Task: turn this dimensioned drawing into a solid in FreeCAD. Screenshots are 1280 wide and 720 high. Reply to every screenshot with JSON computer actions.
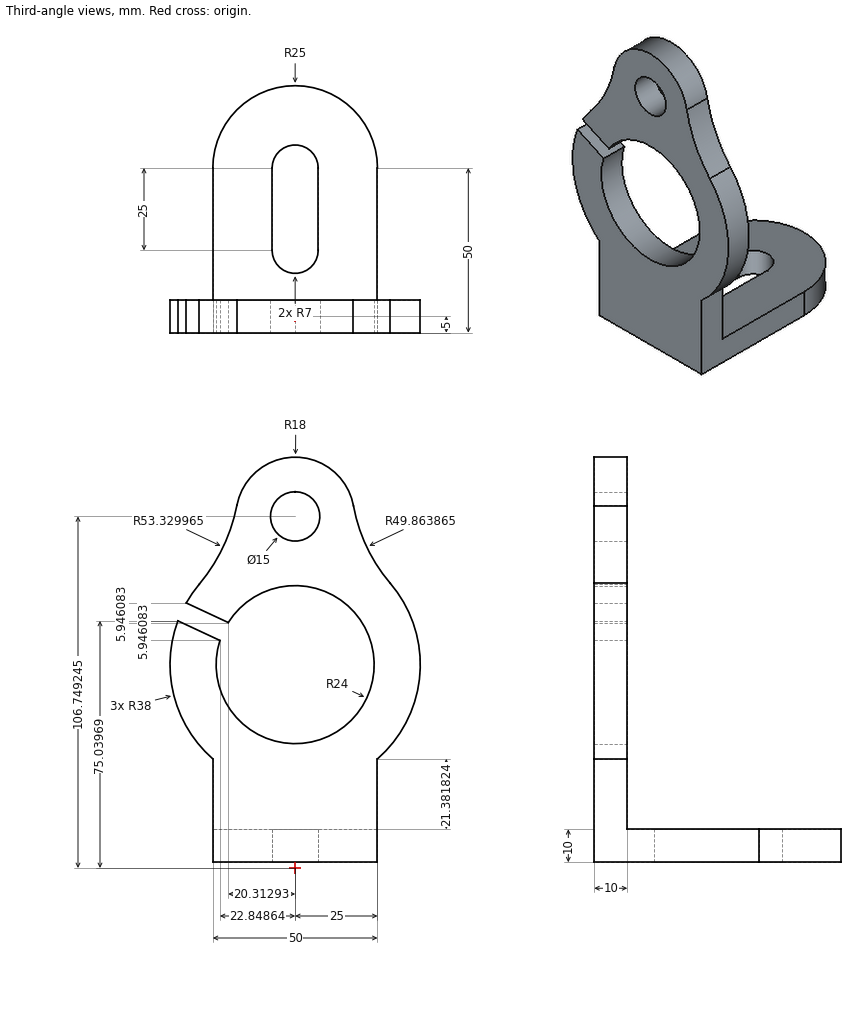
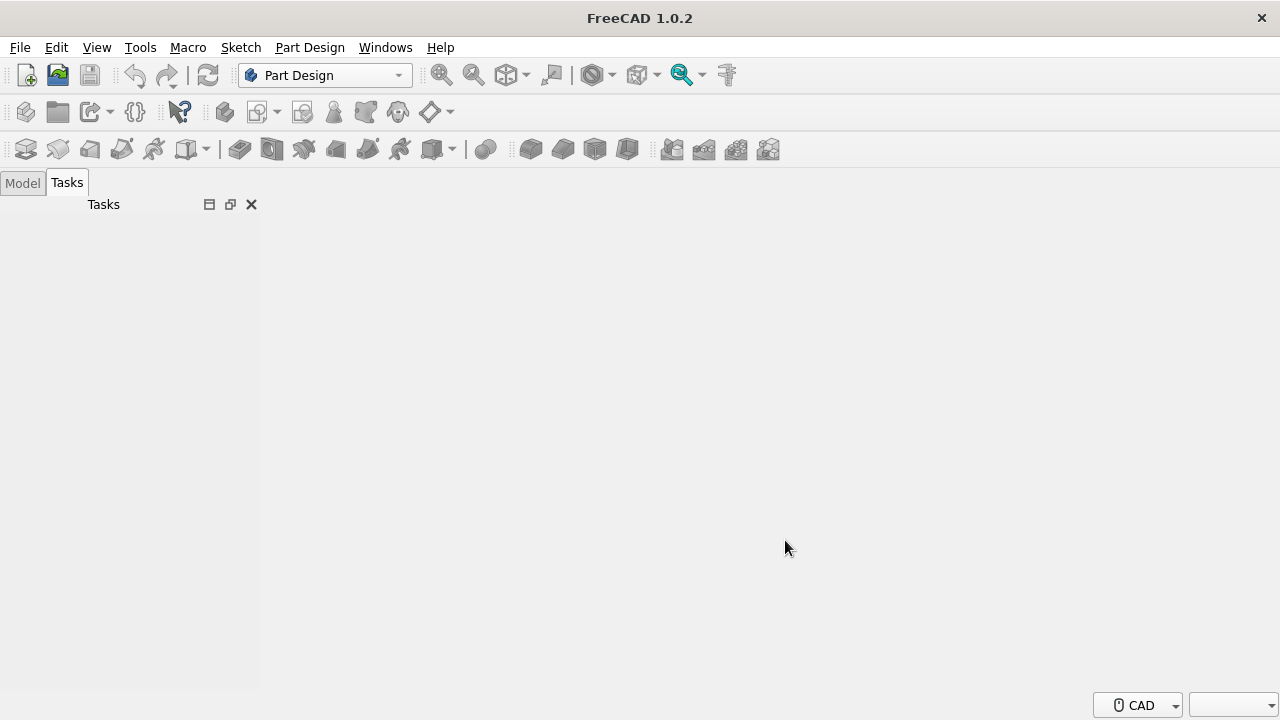
{"action": "left_click", "coordinate": [26, 76]}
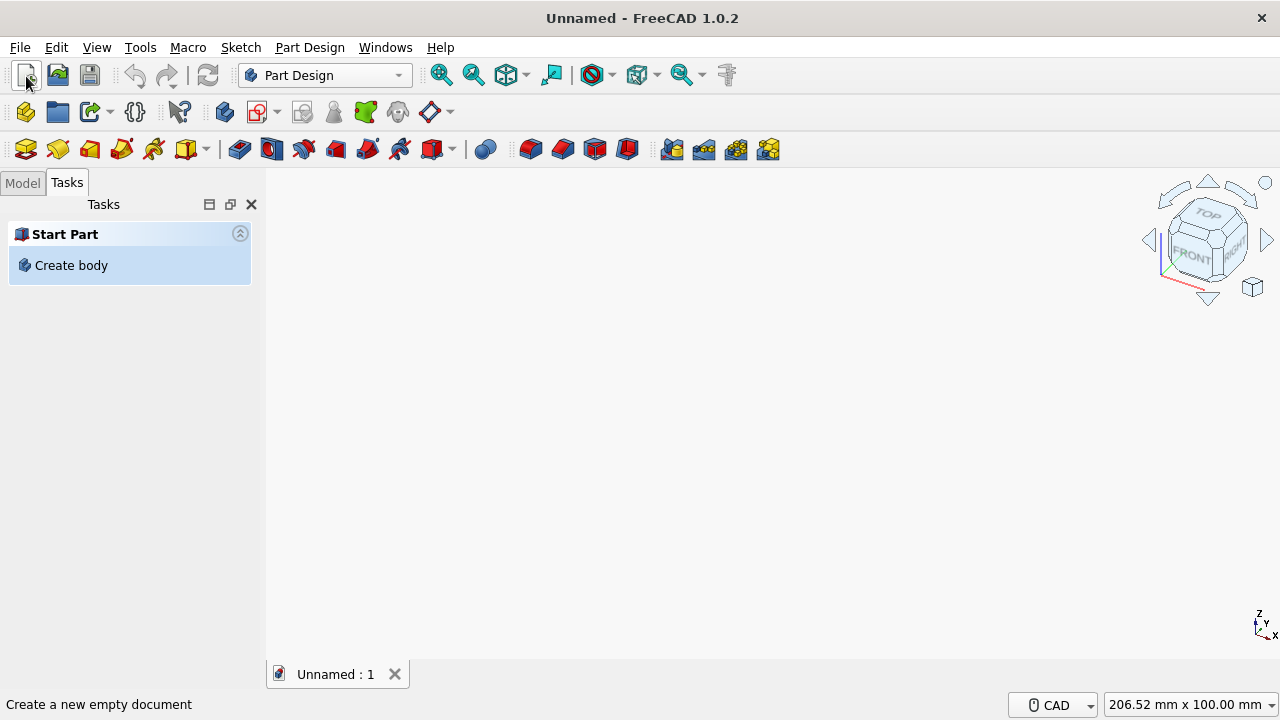
{"action": "left_click", "coordinate": [258, 112]}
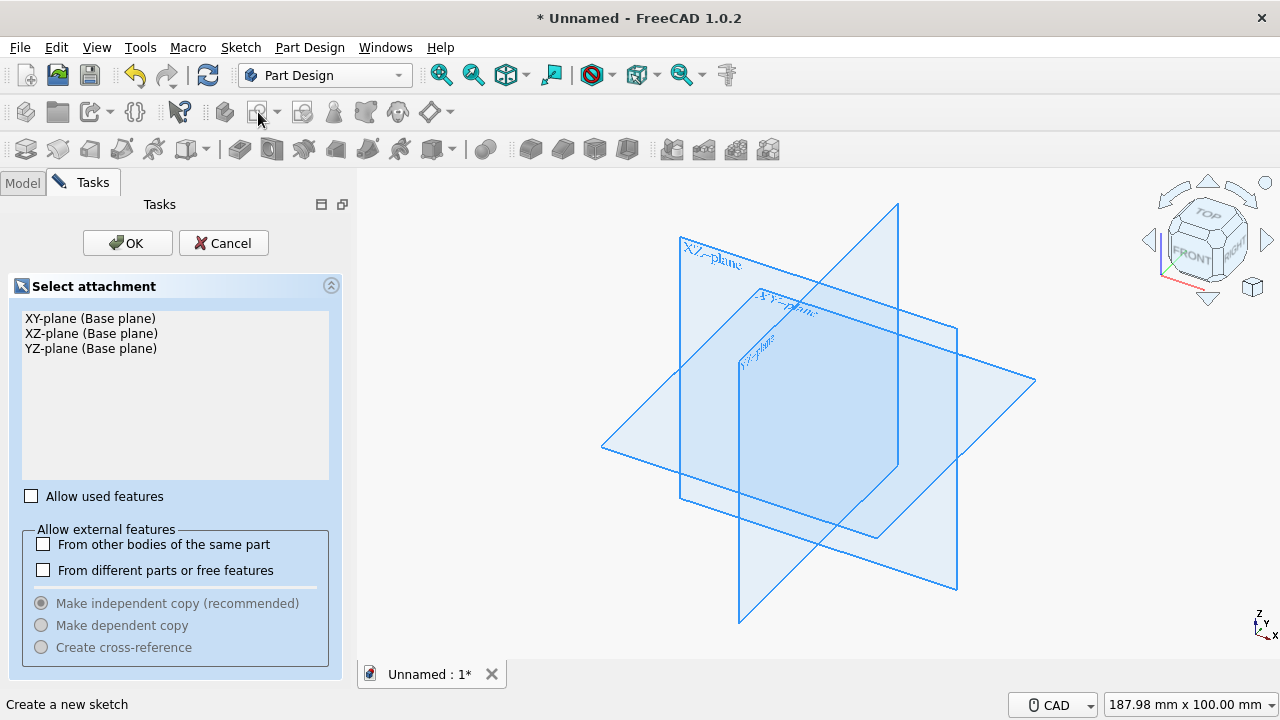
{"action": "left_click", "coordinate": [82, 334]}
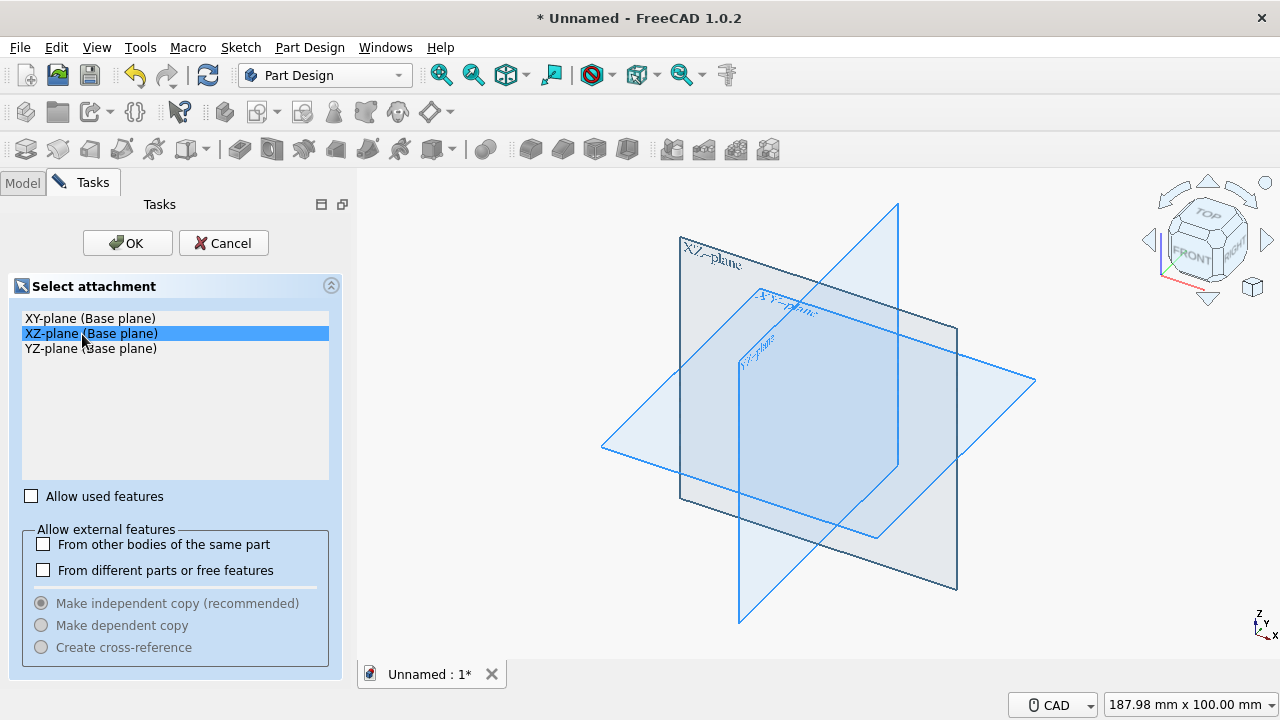
{"action": "left_click", "coordinate": [128, 243]}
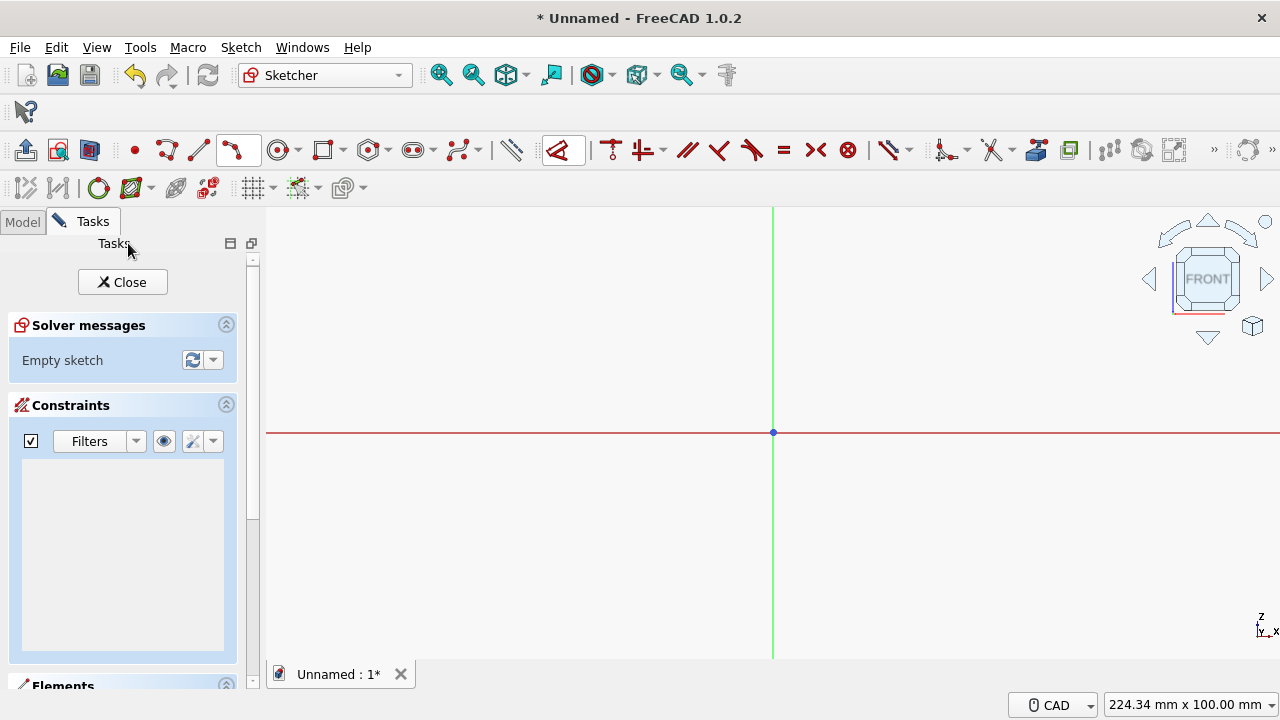
{"action": "scroll", "coordinate": [647, 631], "scroll_direction": "down", "scroll_amount": 4}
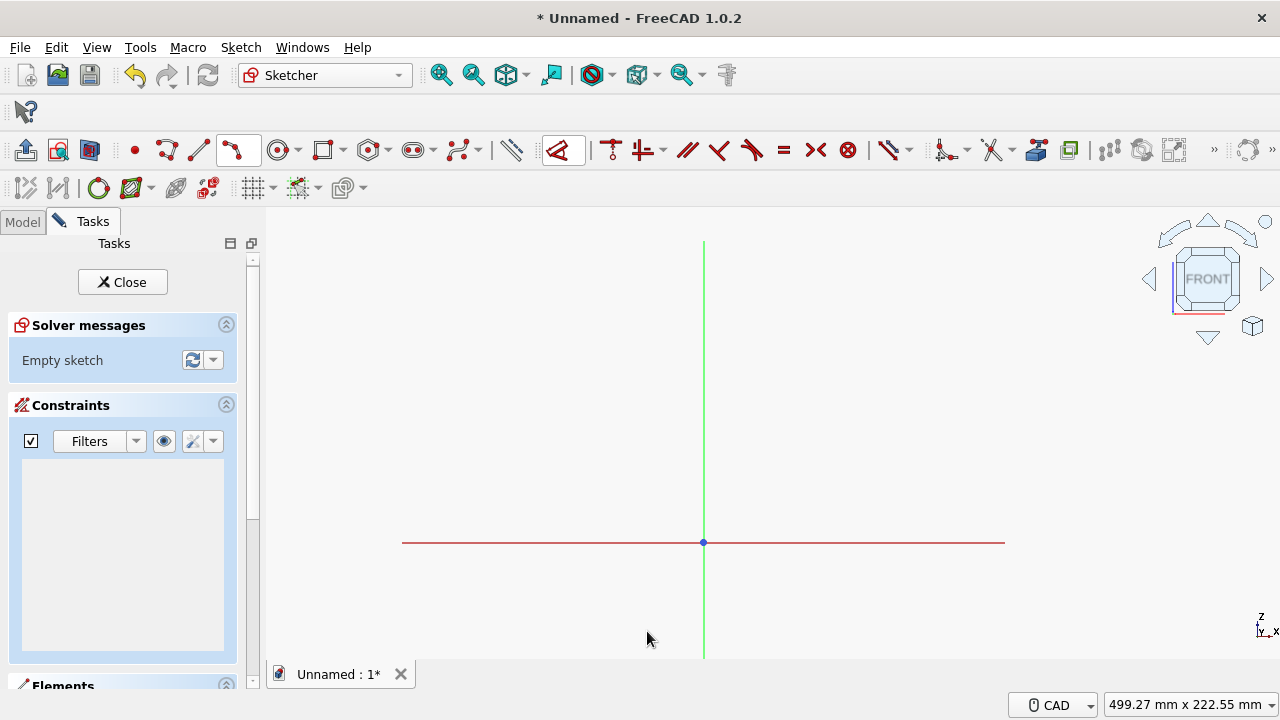
{"action": "left_click", "coordinate": [200, 150]}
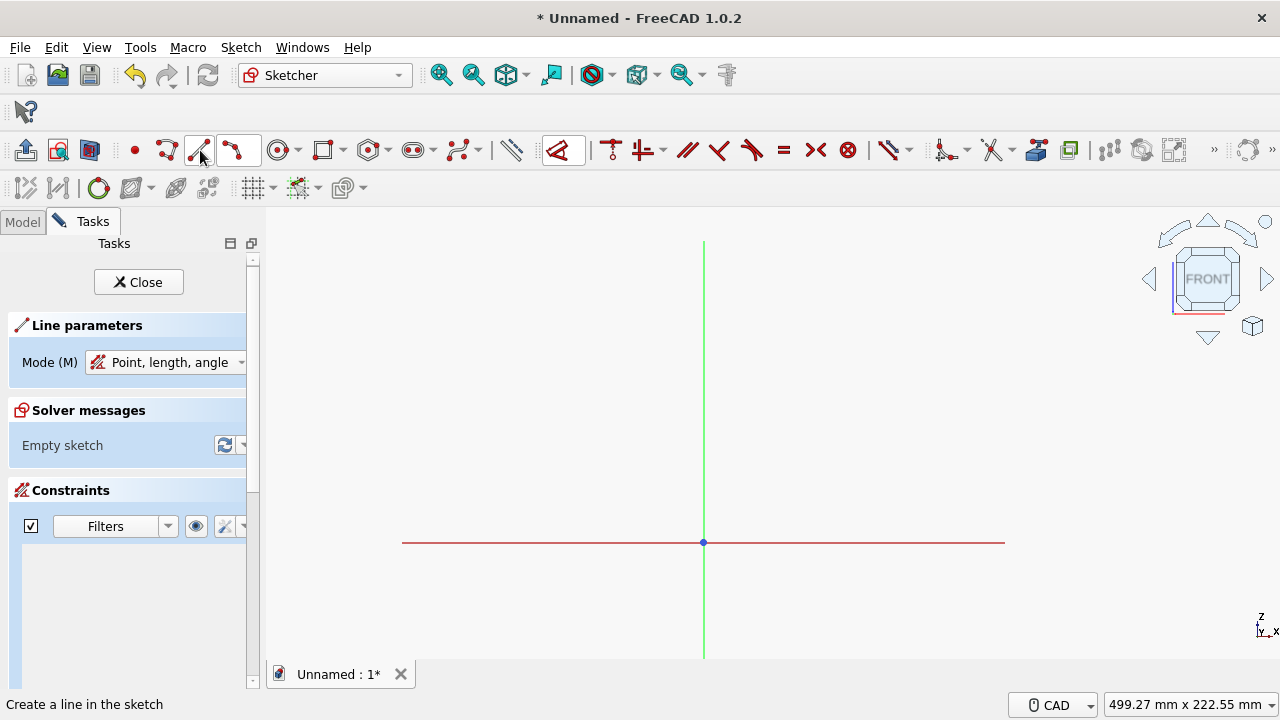
{"action": "left_click", "coordinate": [632, 390]}
{"action": "left_click", "coordinate": [657, 402]}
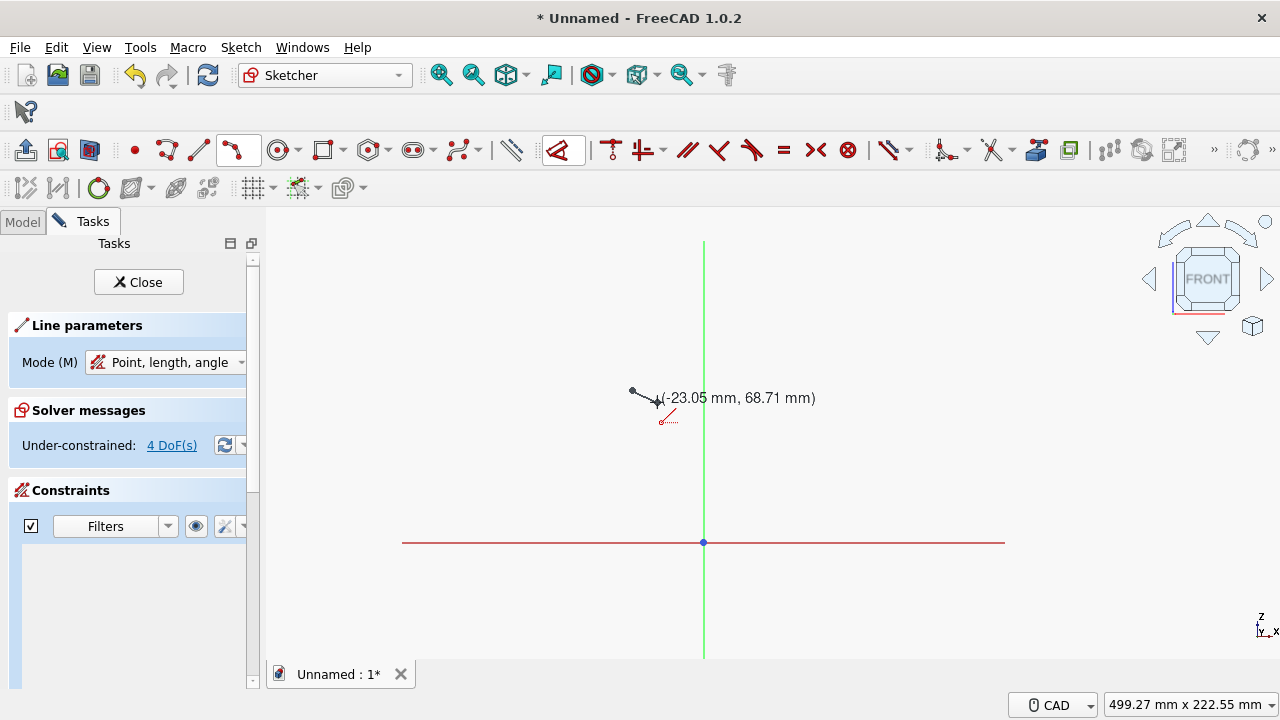
{"action": "scroll", "coordinate": [663, 391], "scroll_direction": "up", "scroll_amount": 2}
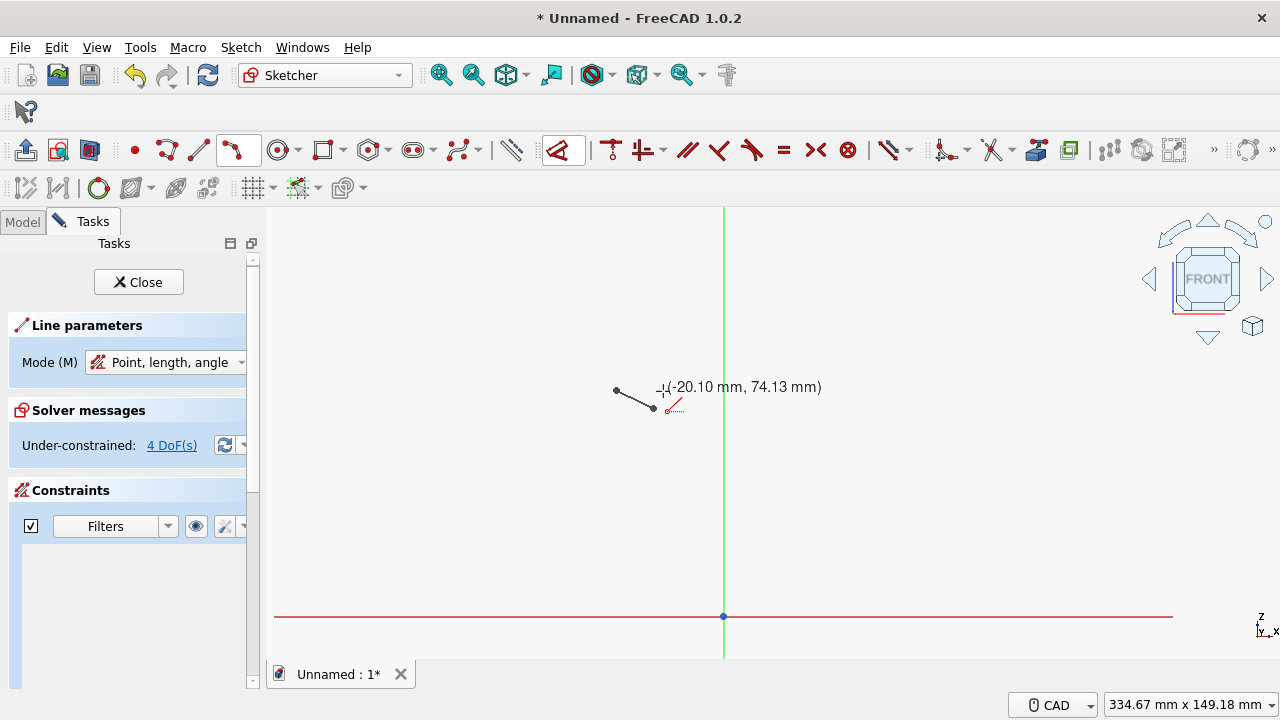
{"action": "left_click", "coordinate": [662, 391]}
{"action": "left_click", "coordinate": [624, 373]}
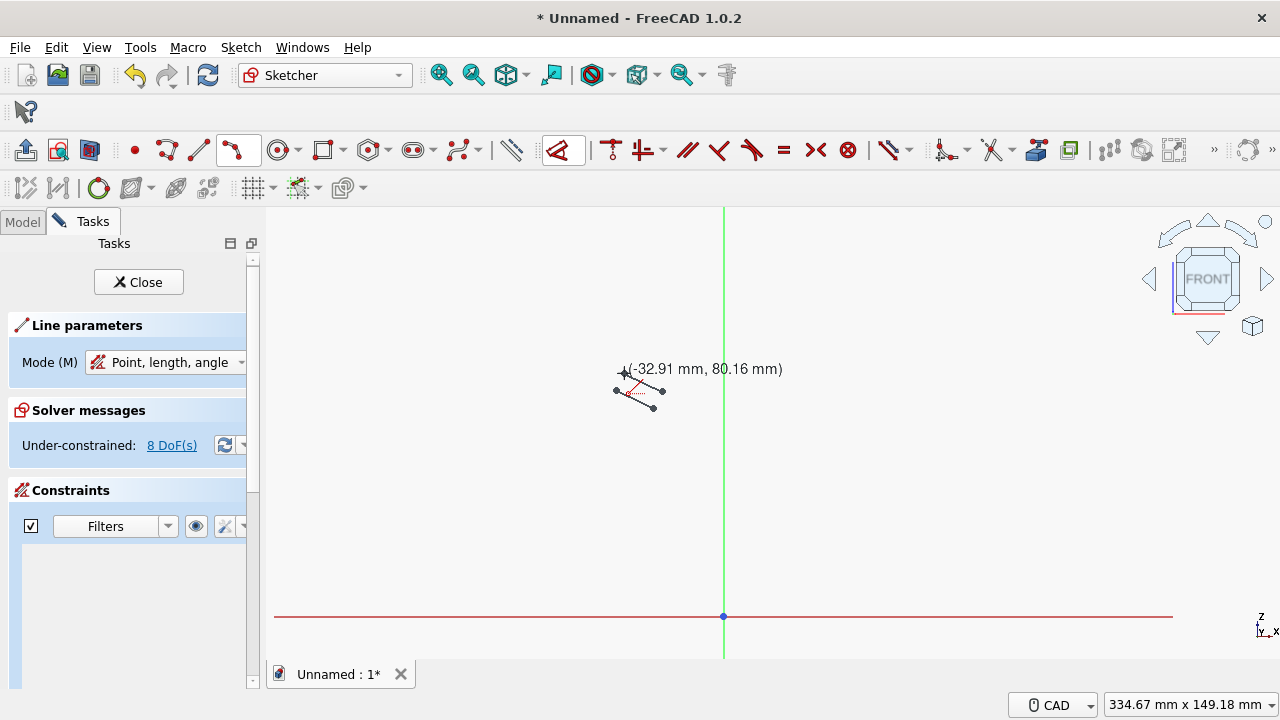
{"action": "left_click", "coordinate": [168, 150]}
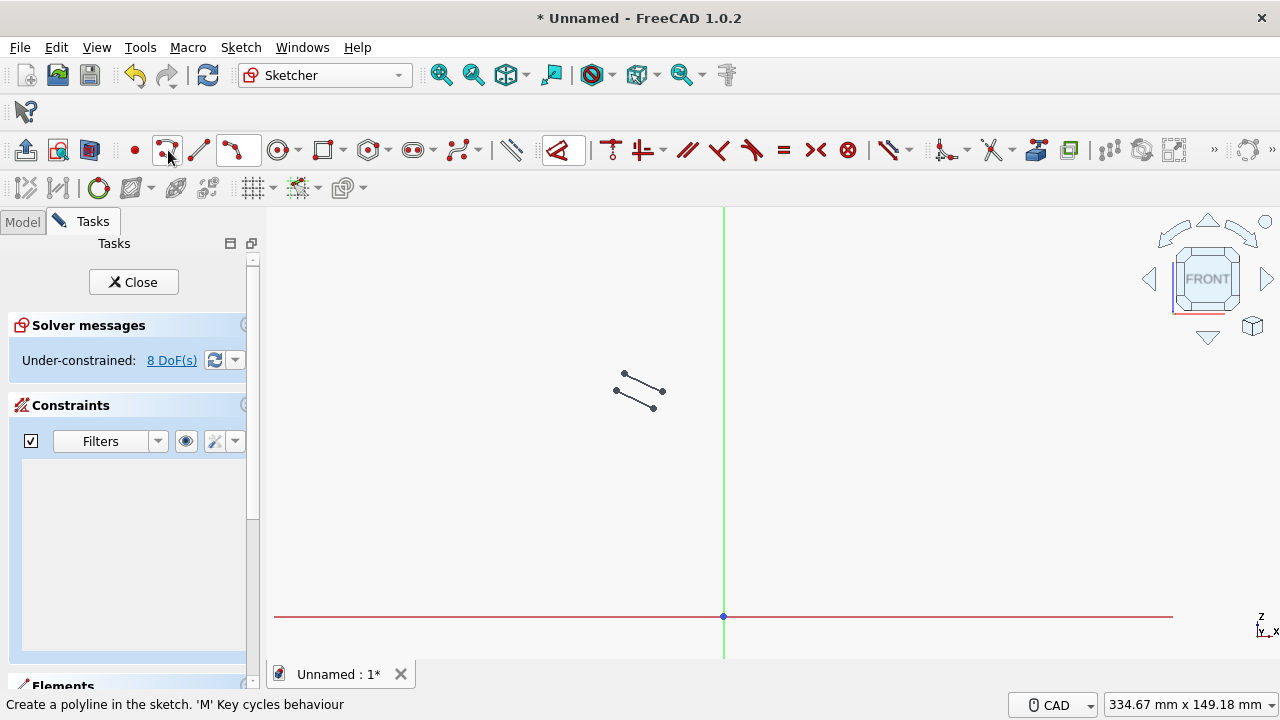
{"action": "left_click", "coordinate": [799, 517]}
{"action": "left_click", "coordinate": [799, 581]}
{"action": "left_click", "coordinate": [648, 581]}
{"action": "left_click", "coordinate": [648, 517]}
{"action": "right_click", "coordinate": [648, 517]}